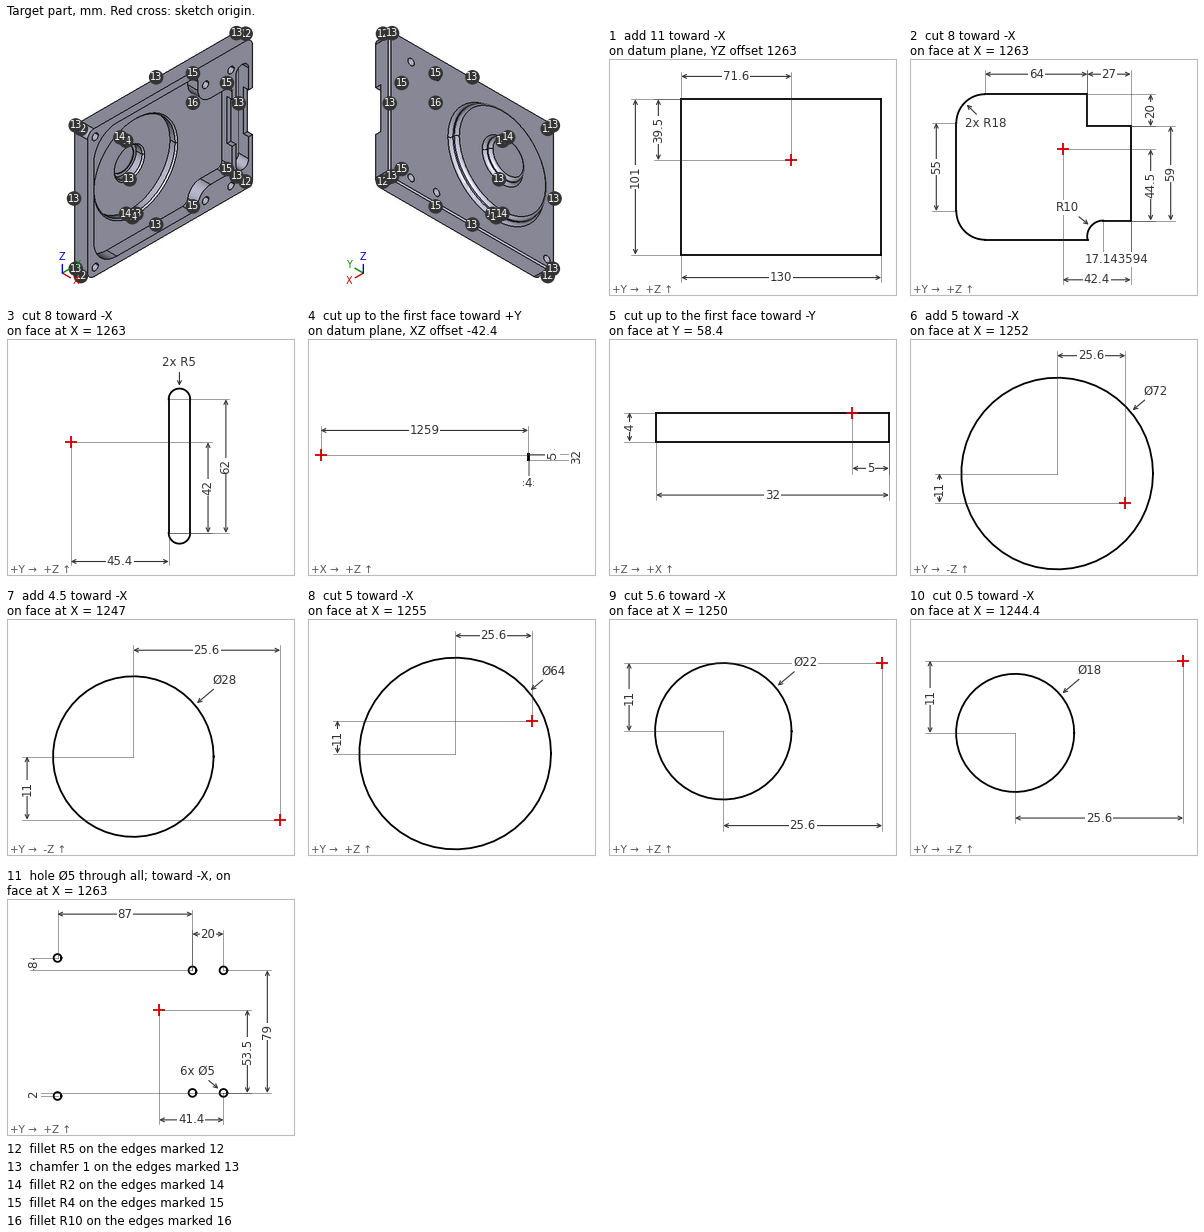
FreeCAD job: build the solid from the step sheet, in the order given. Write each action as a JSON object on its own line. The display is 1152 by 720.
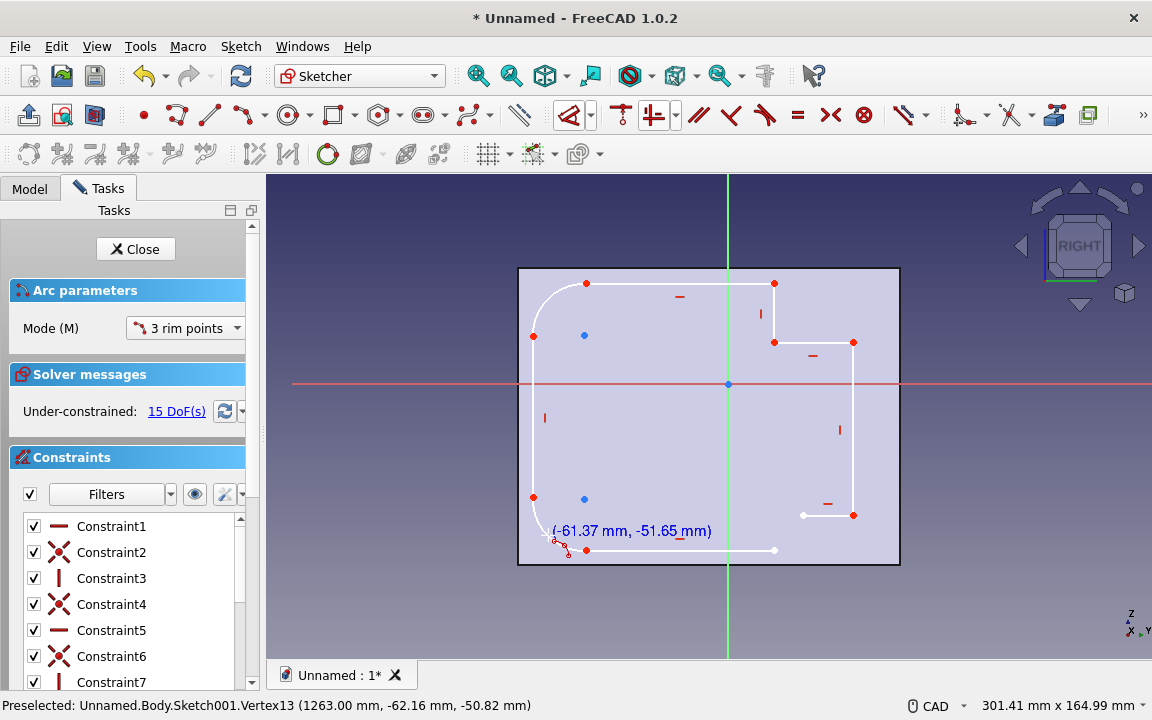
{"action": "left_click", "coordinate": [774, 551]}
{"action": "left_click", "coordinate": [803, 516]}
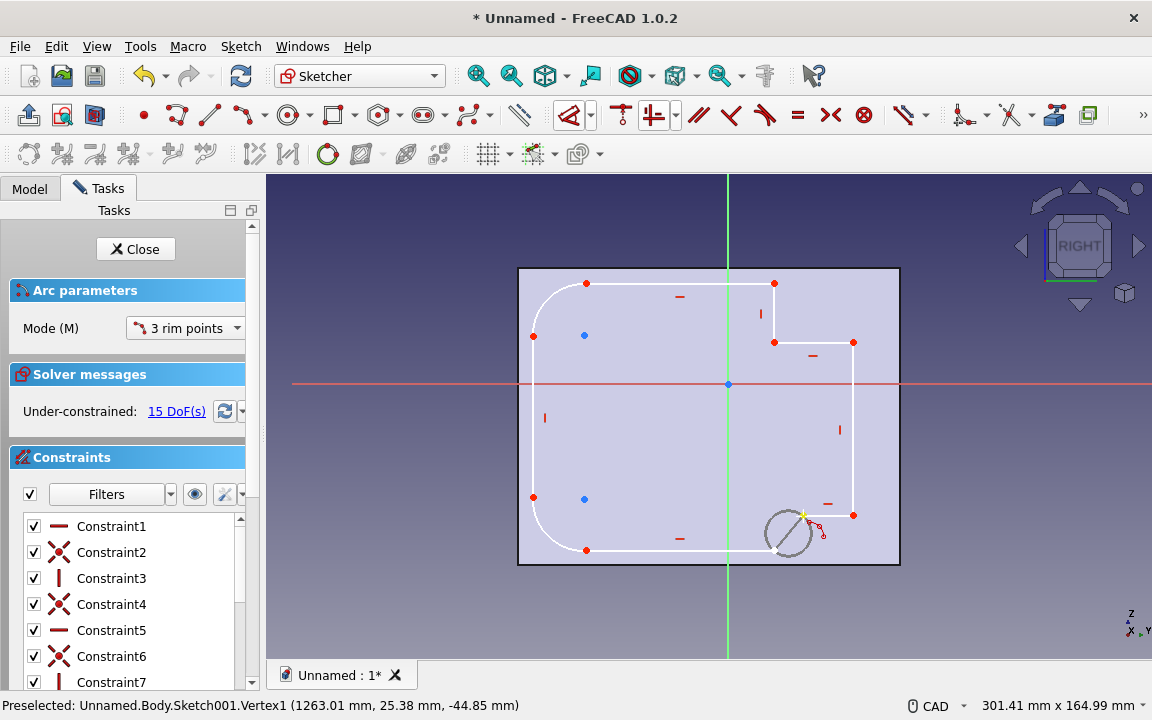
{"action": "scroll", "coordinate": [780, 526], "scroll_direction": "up", "scroll_amount": 2}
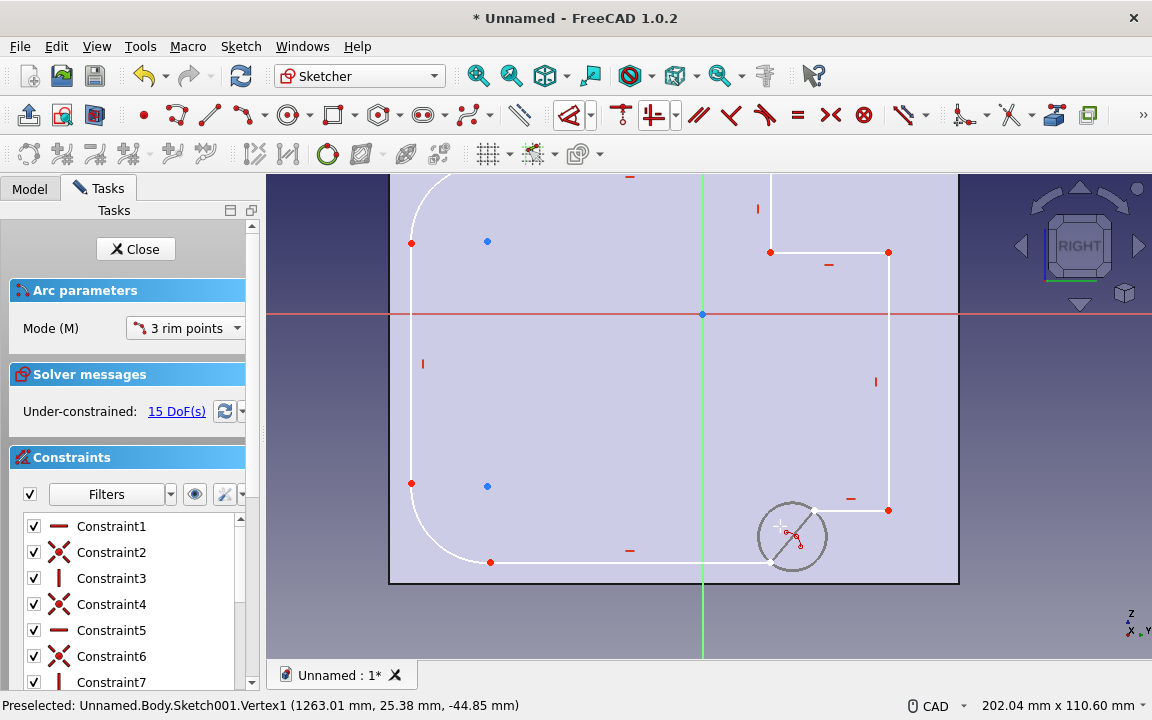
{"action": "left_click", "coordinate": [780, 525]}
{"action": "key", "text": "Escape"}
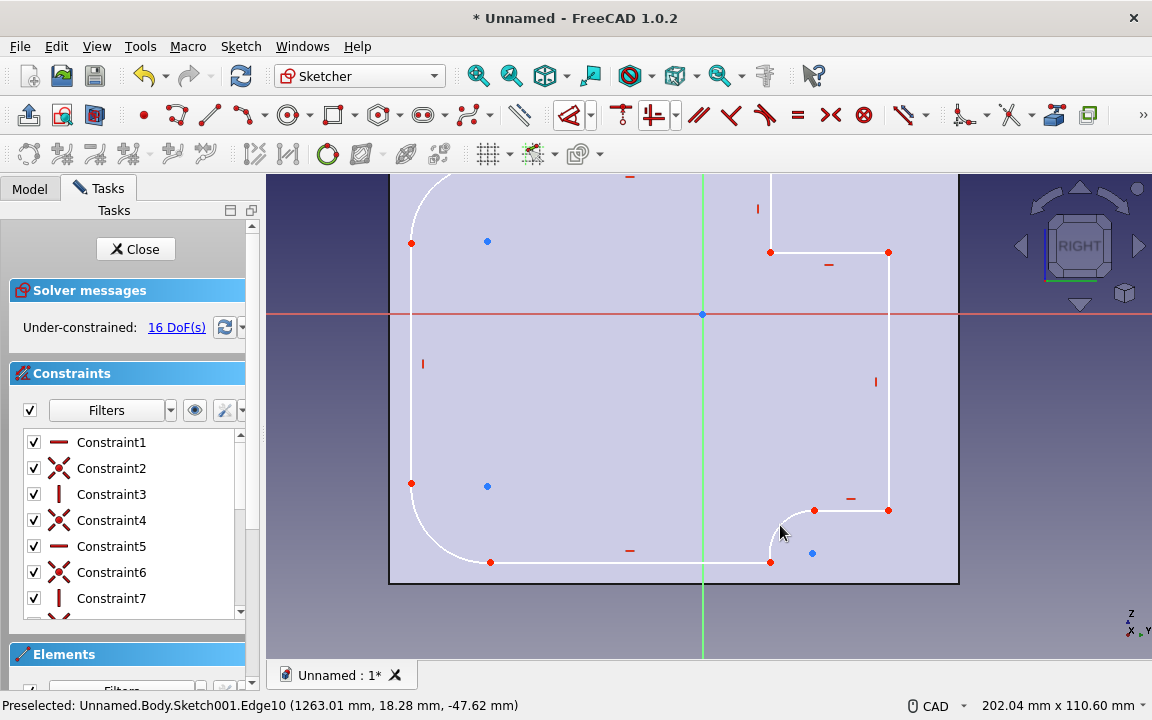
{"action": "left_click", "coordinate": [836, 511]}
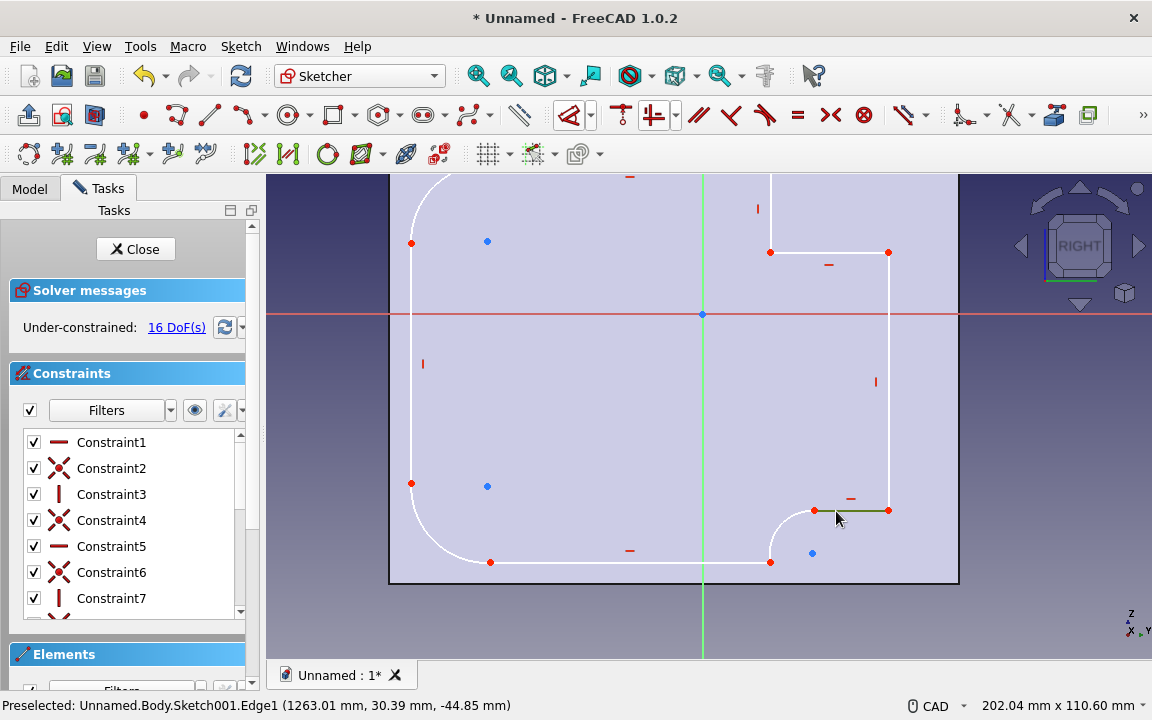
{"action": "left_click", "coordinate": [792, 516]}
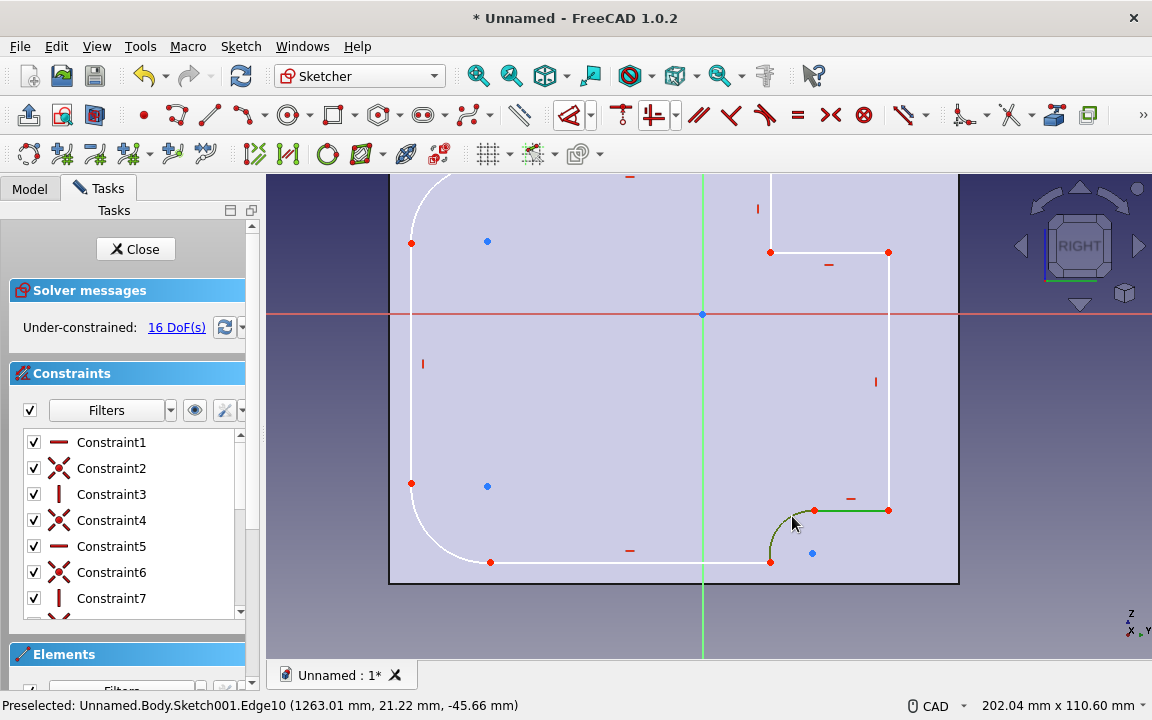
{"action": "left_click", "coordinate": [765, 116]}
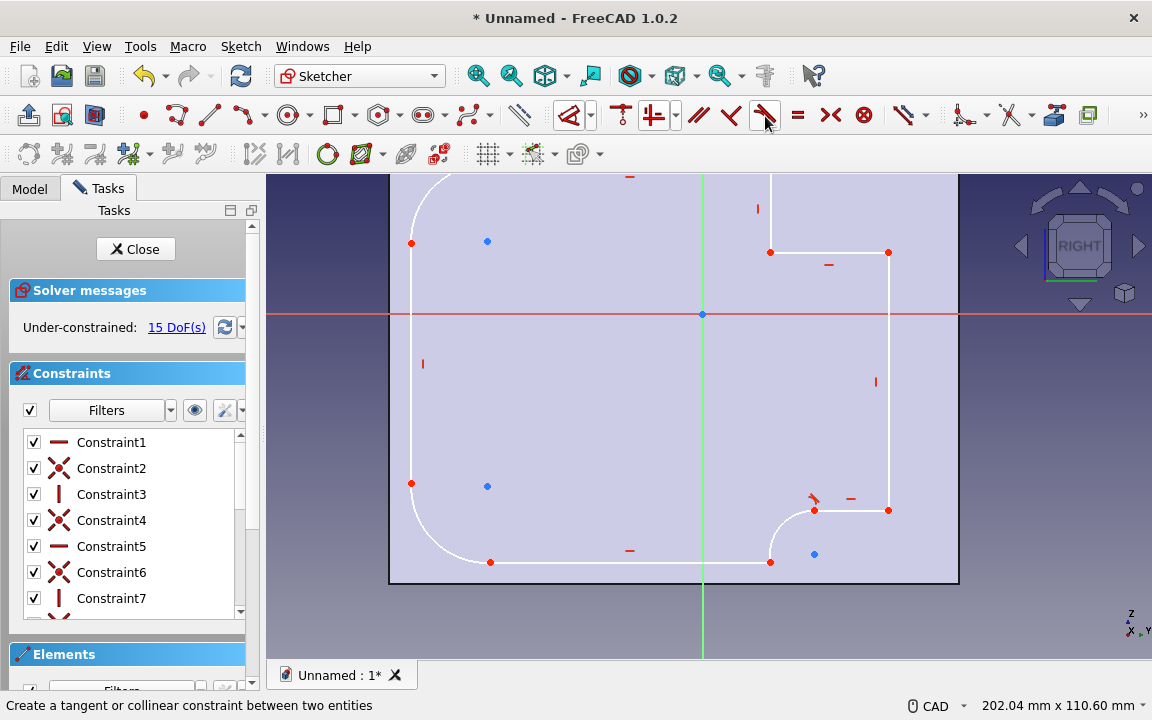
{"action": "scroll", "coordinate": [599, 631], "scroll_direction": "down", "scroll_amount": 1}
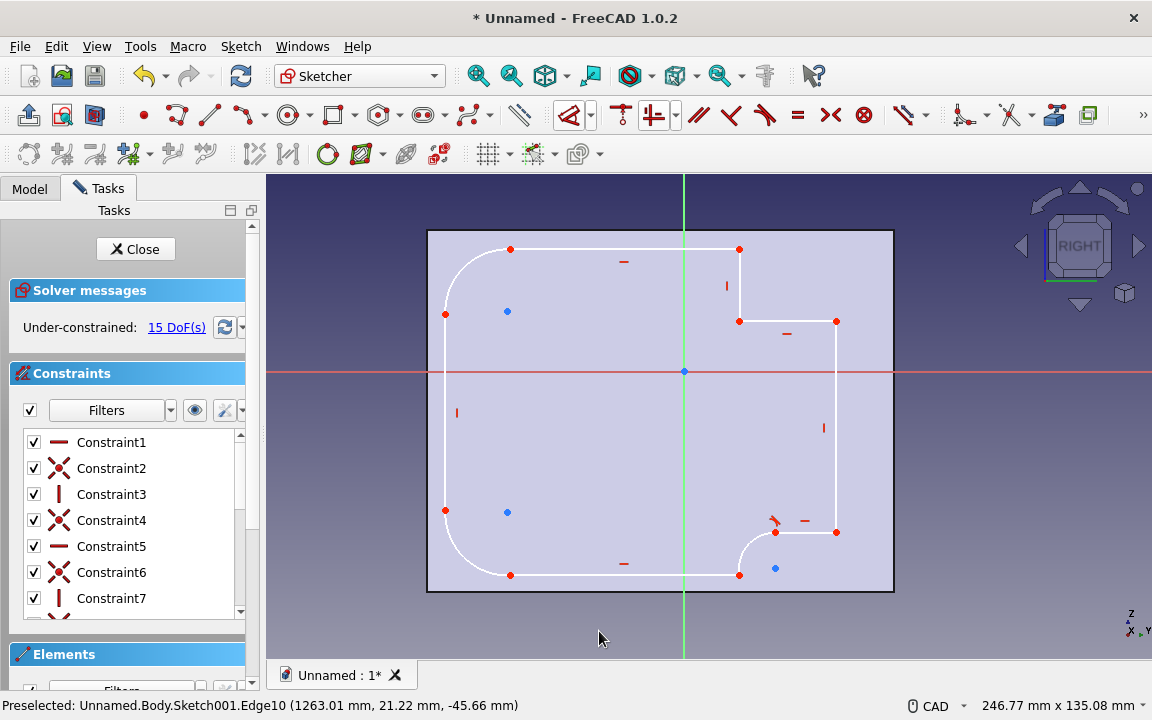
{"action": "left_click", "coordinate": [671, 249]}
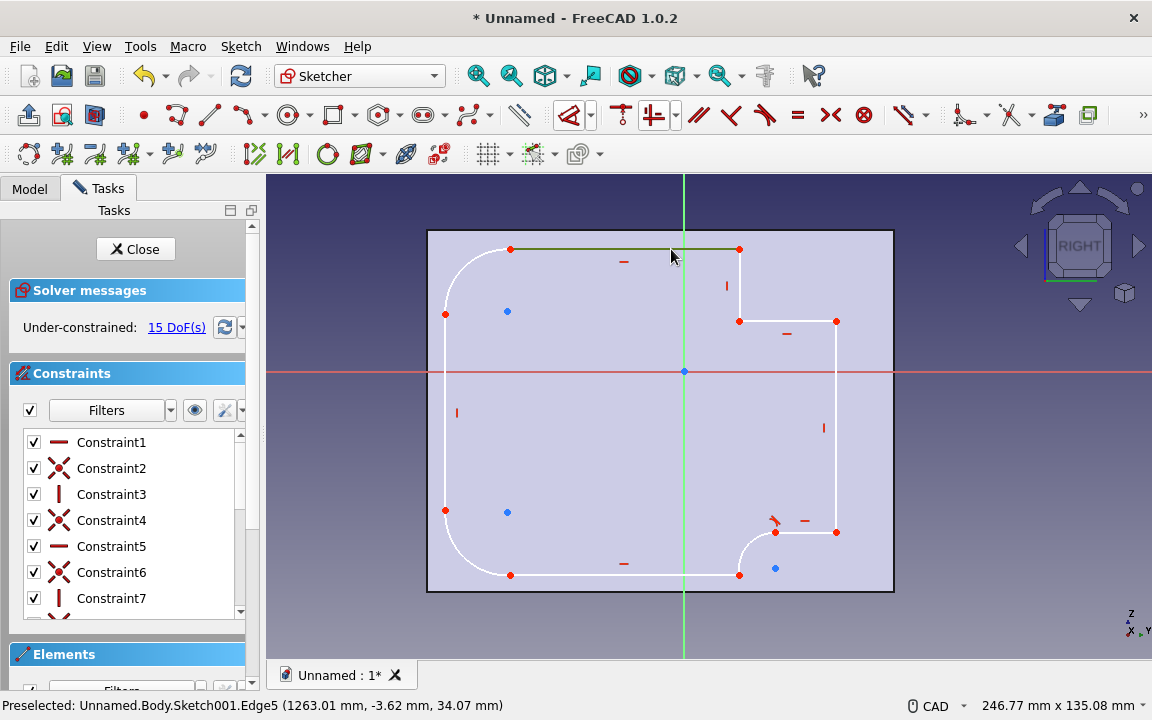
{"action": "left_click", "coordinate": [480, 256]}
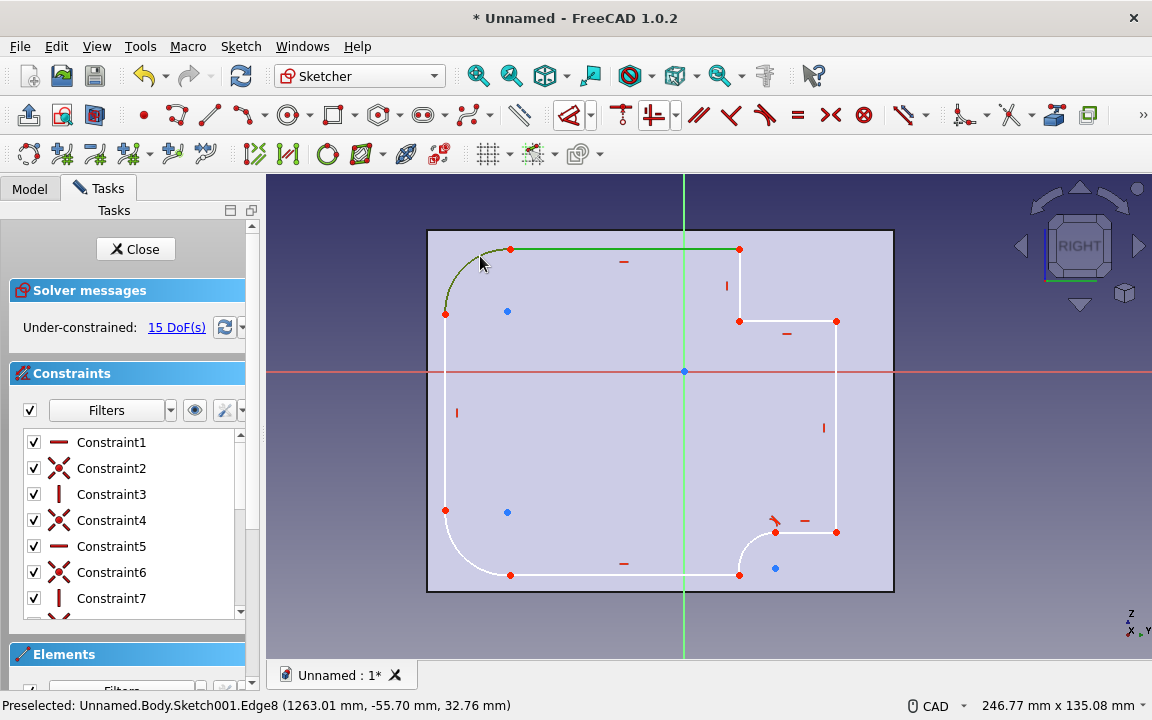
{"action": "left_click", "coordinate": [765, 116]}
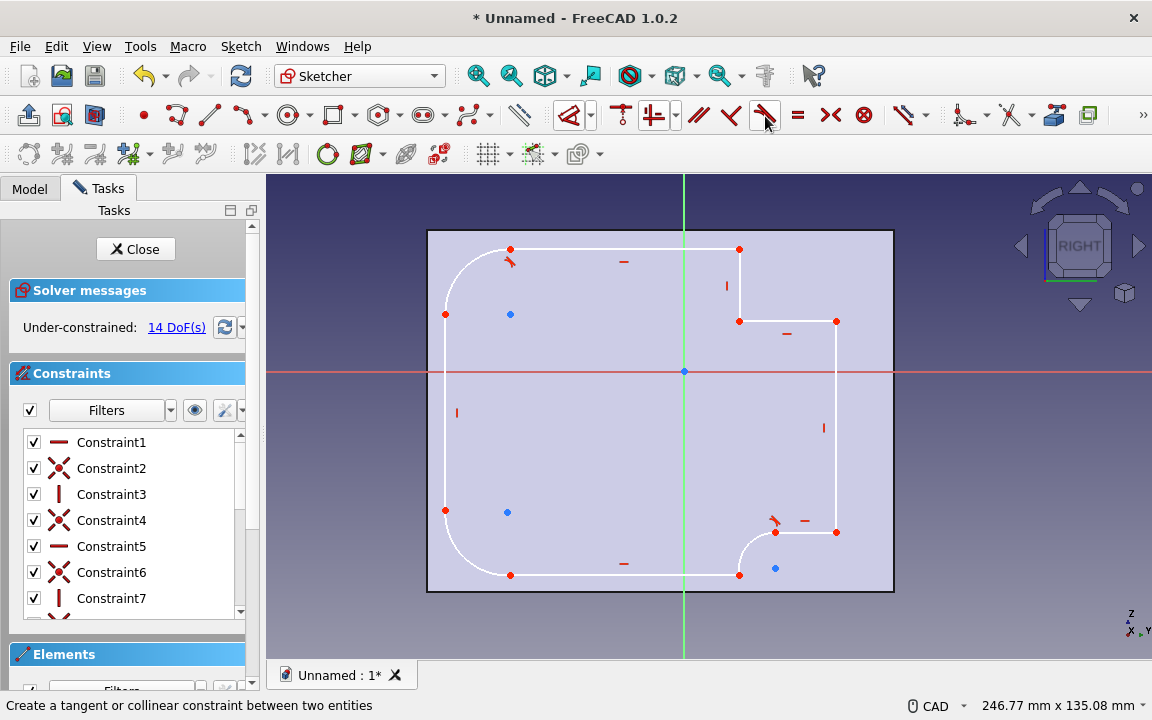
{"action": "left_click", "coordinate": [445, 373]}